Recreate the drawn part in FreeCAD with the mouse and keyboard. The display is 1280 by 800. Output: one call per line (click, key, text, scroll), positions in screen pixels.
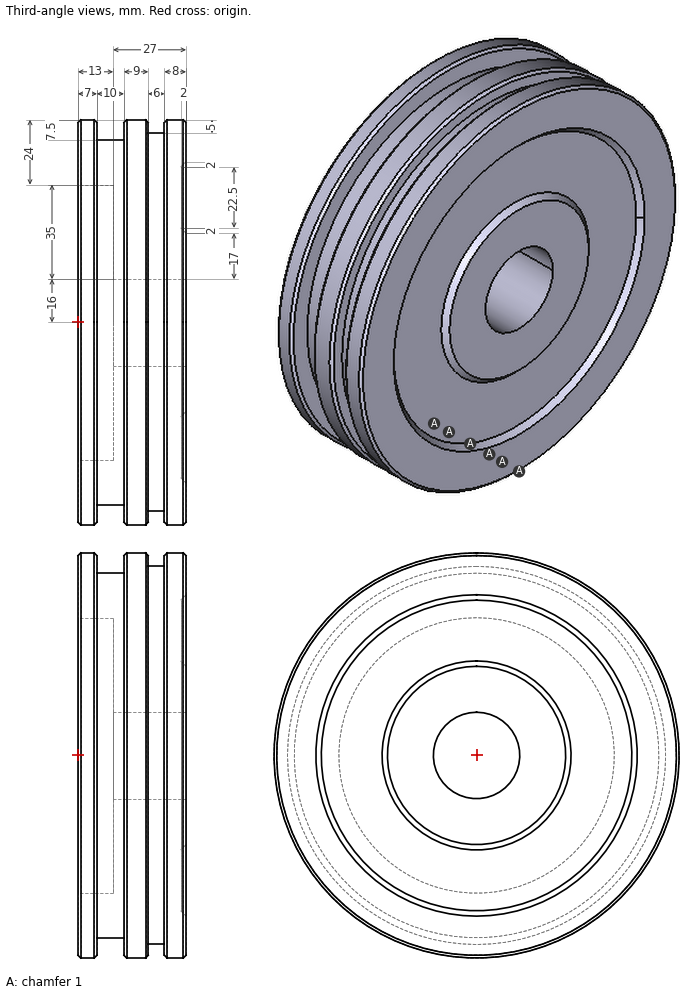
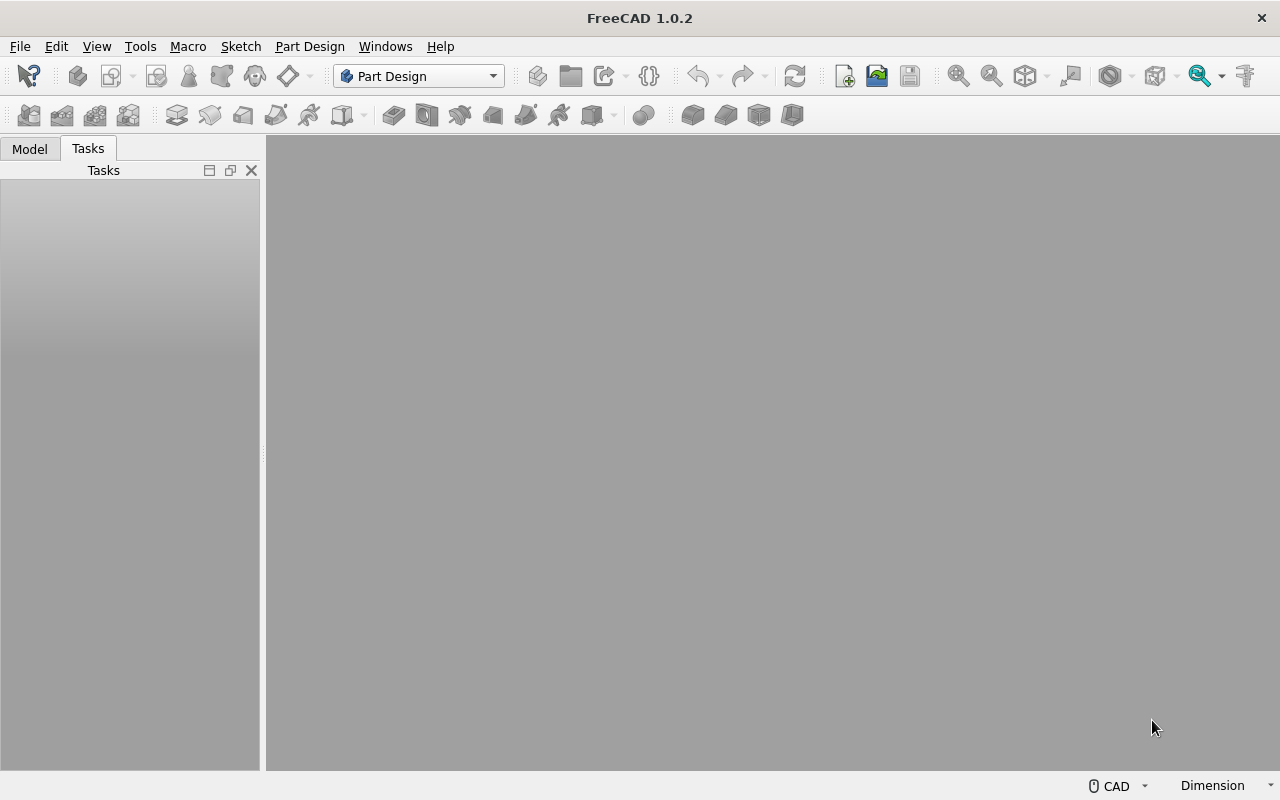
click(844, 76)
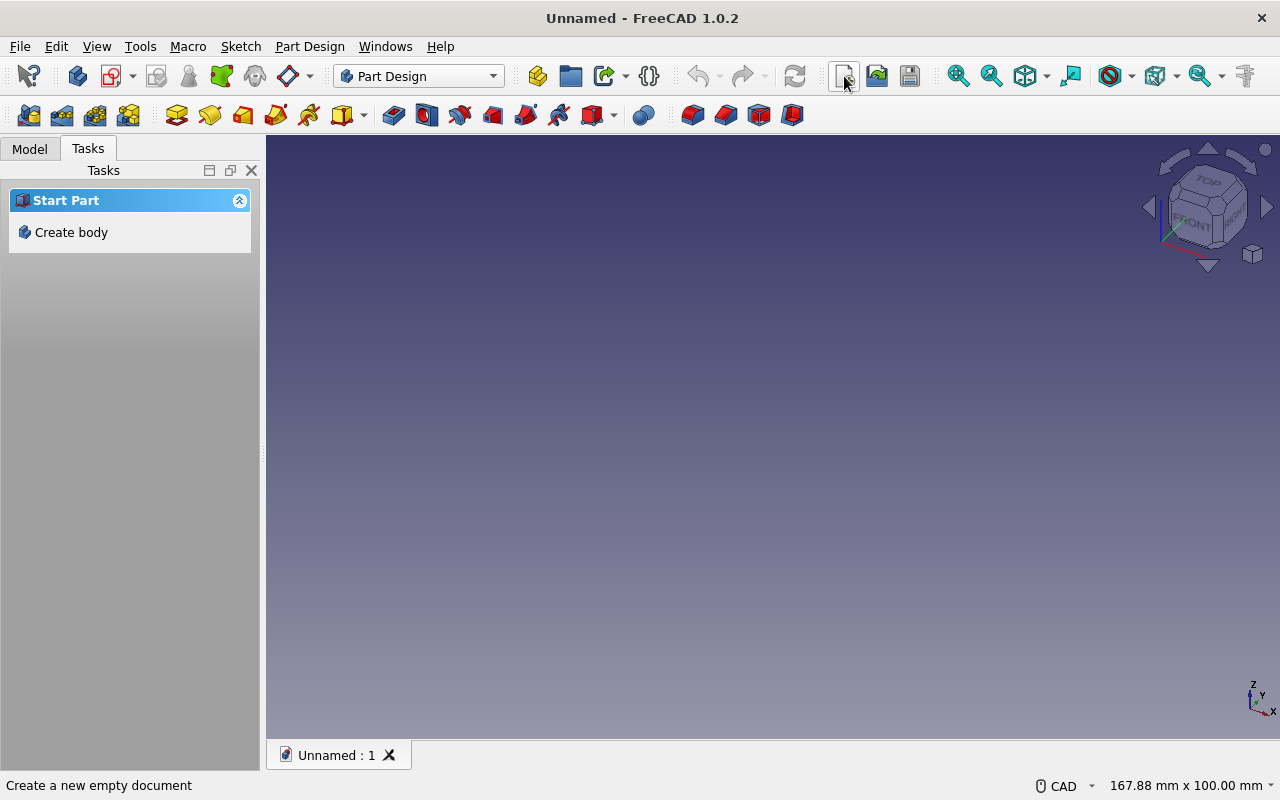
click(110, 76)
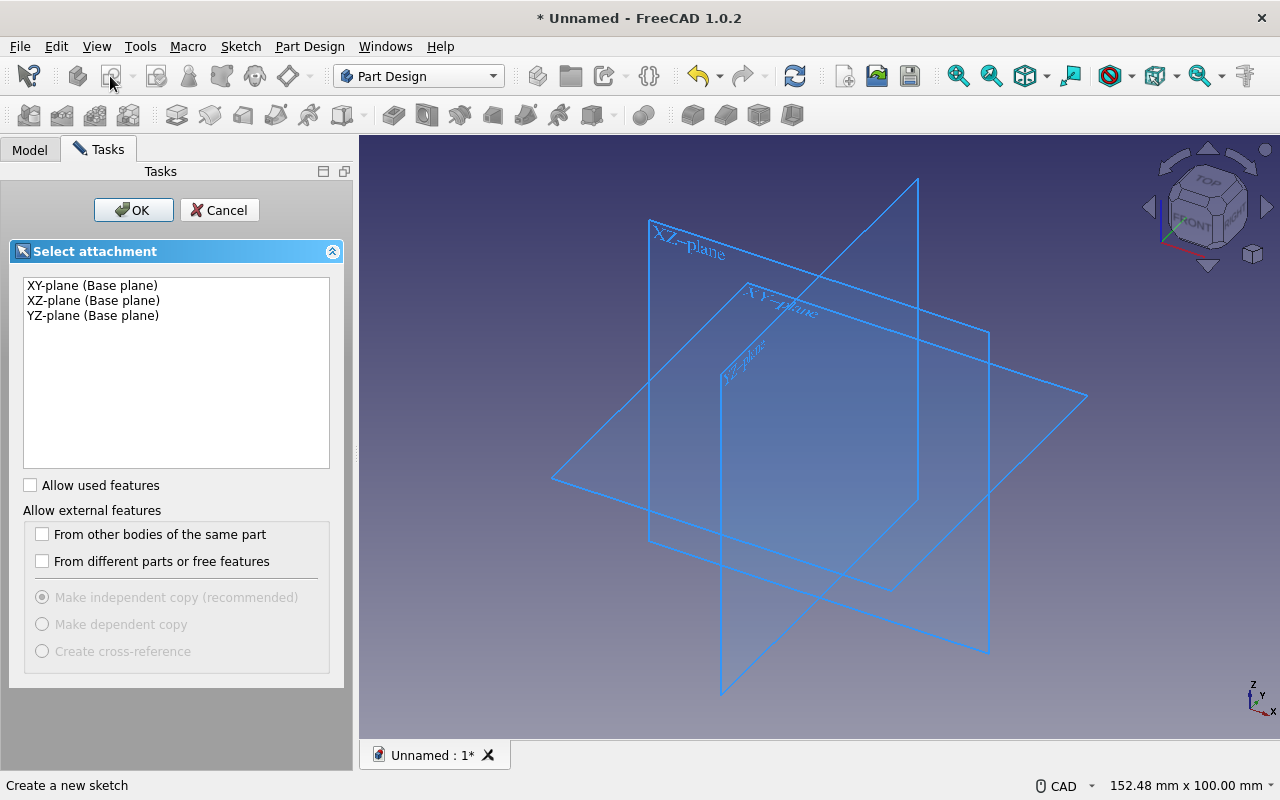
click(84, 286)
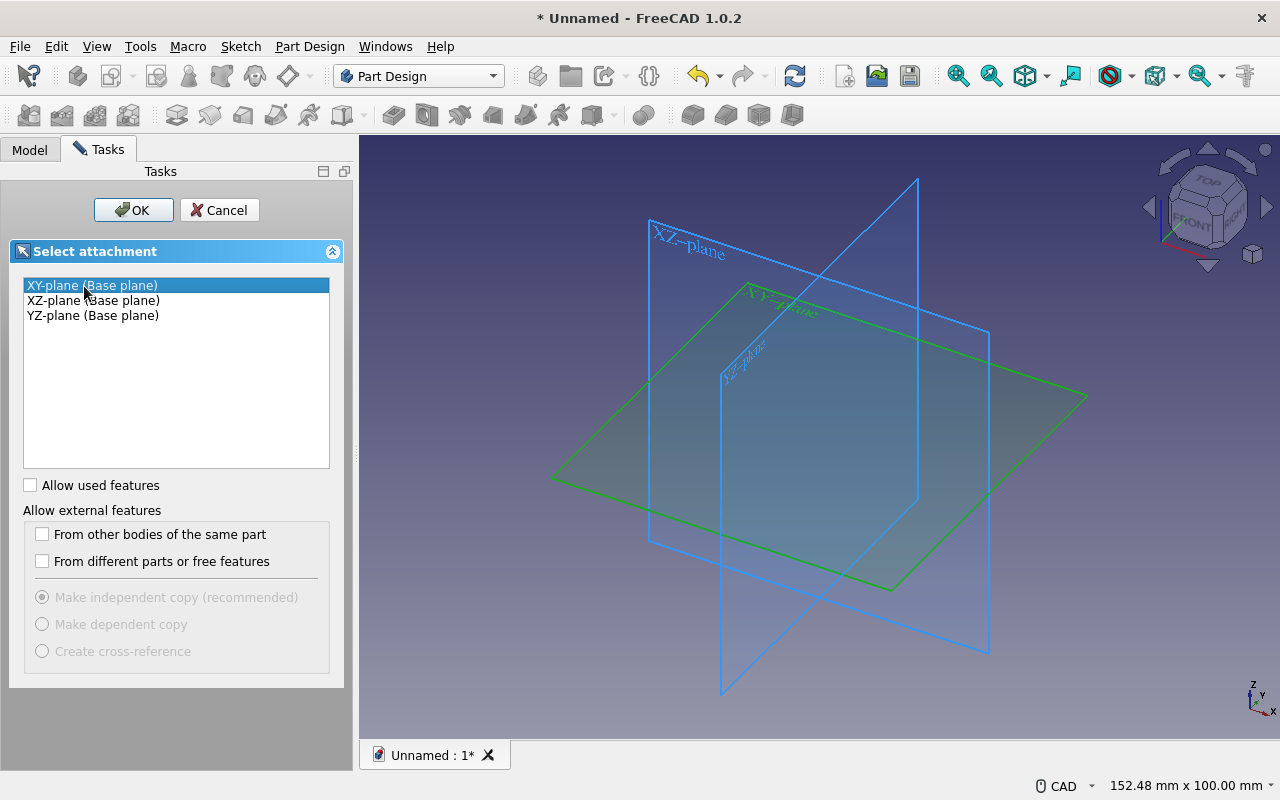
click(134, 210)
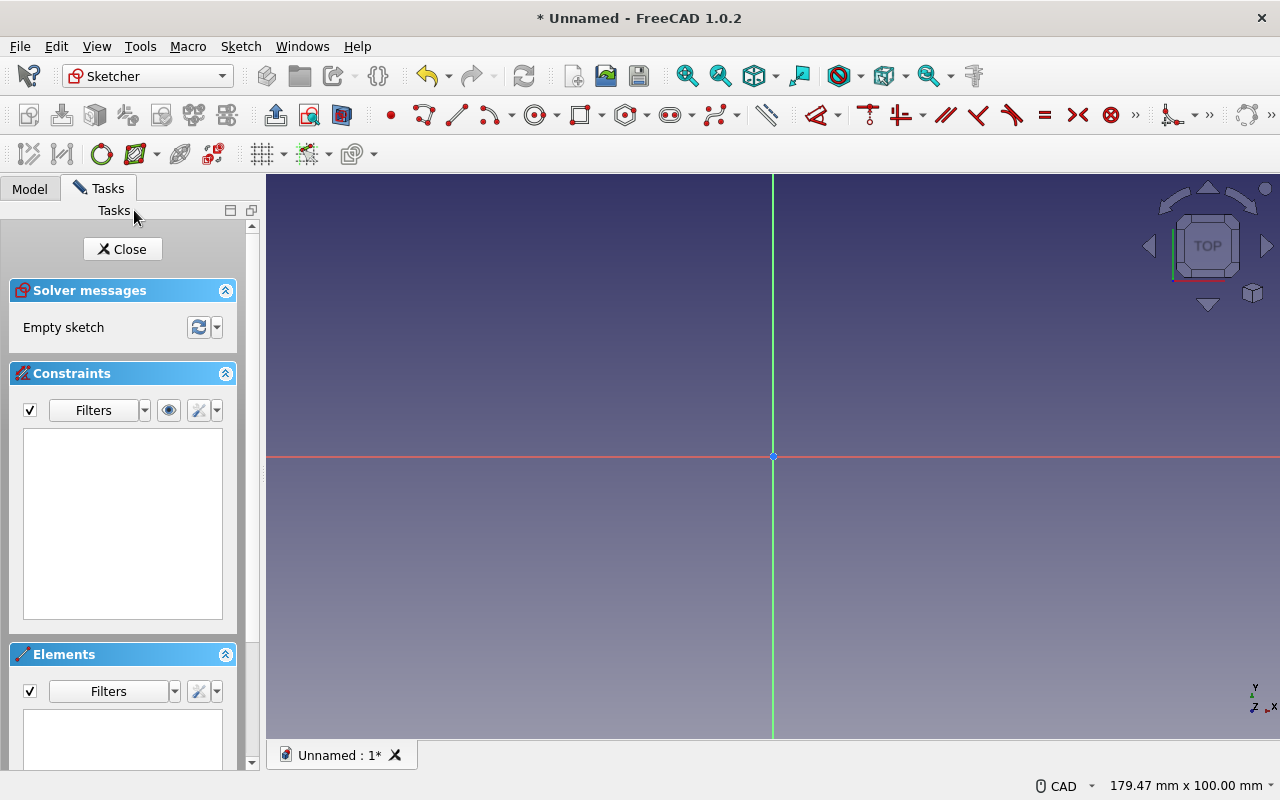
scroll(335, 711, down, 2)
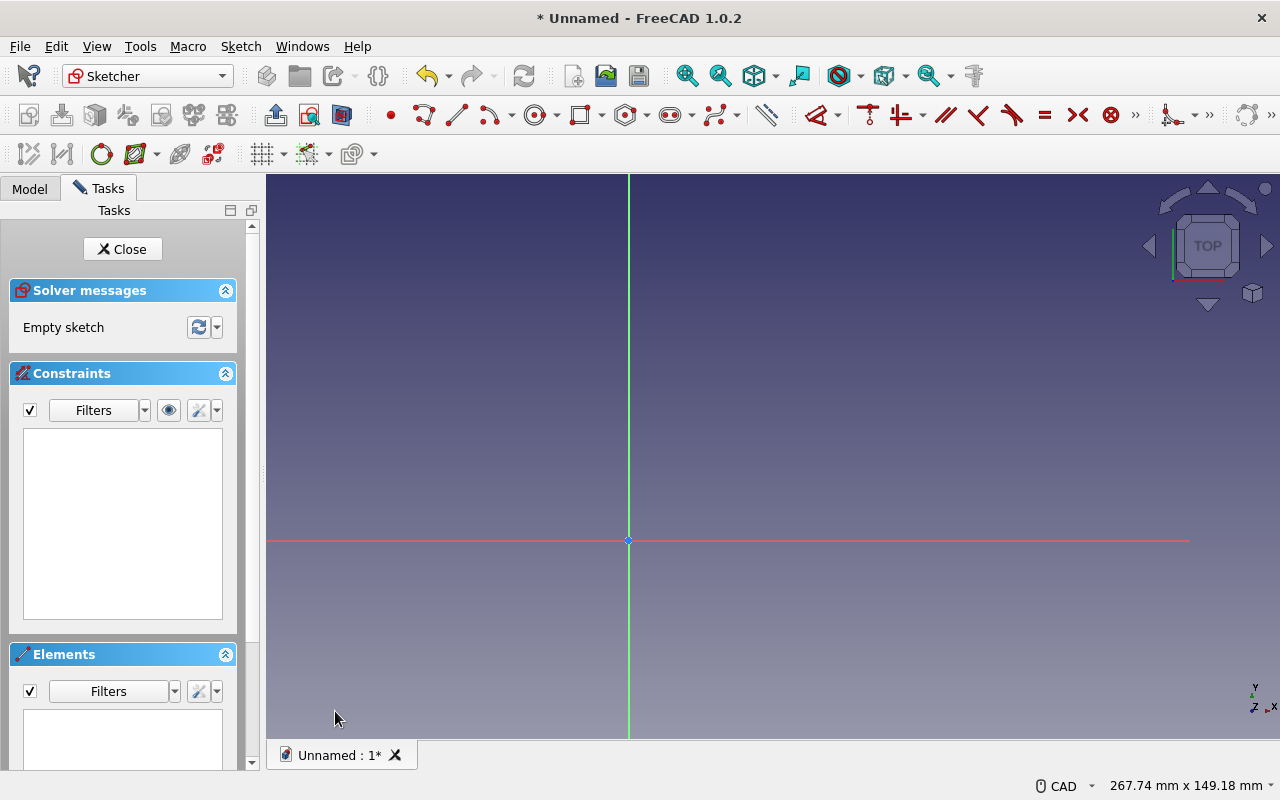
click(424, 116)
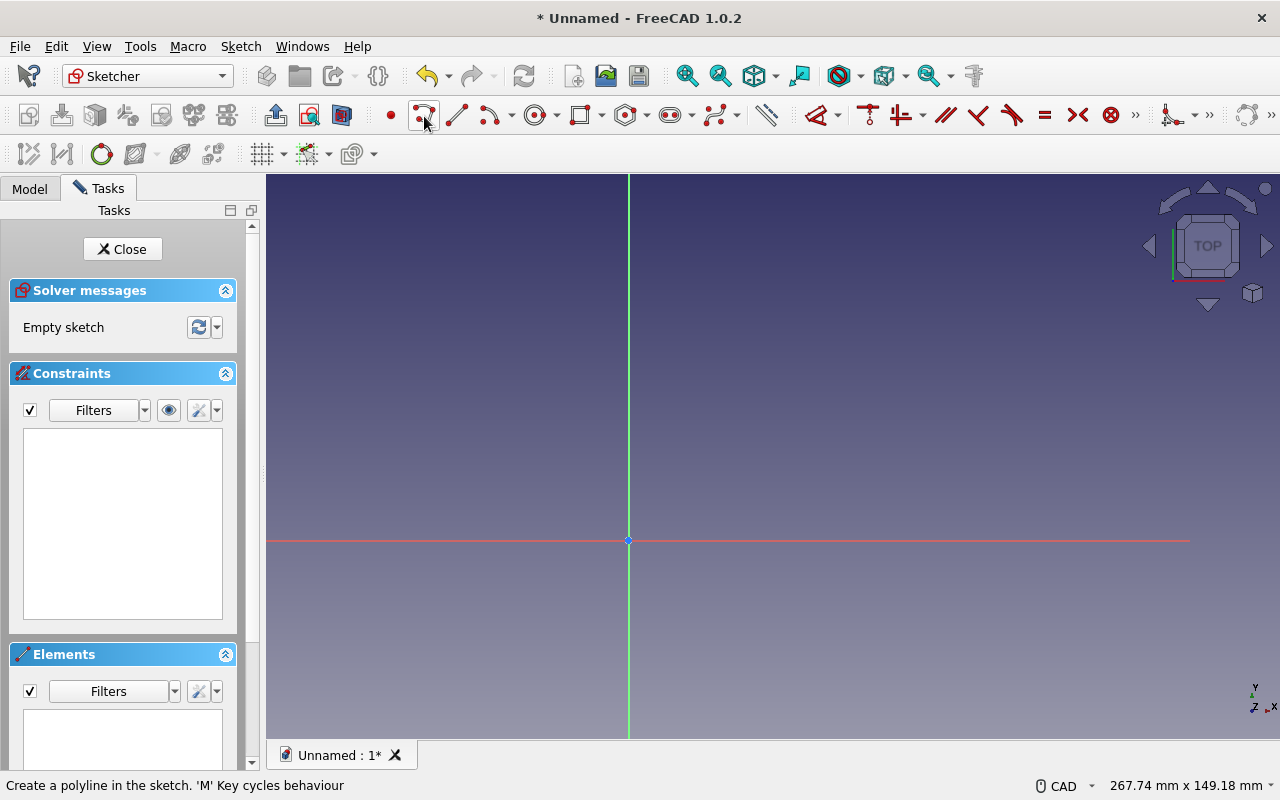
click(678, 480)
click(780, 480)
click(780, 416)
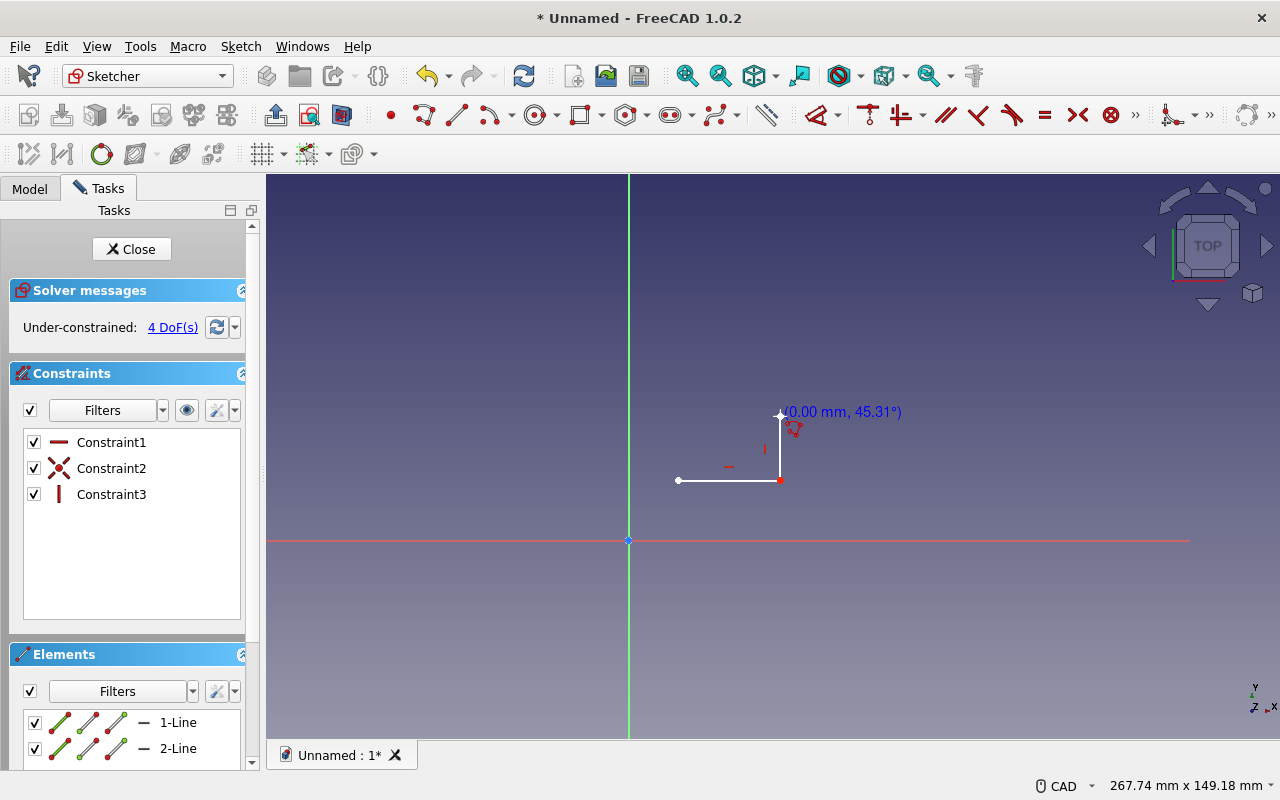
scroll(773, 408, up, 2)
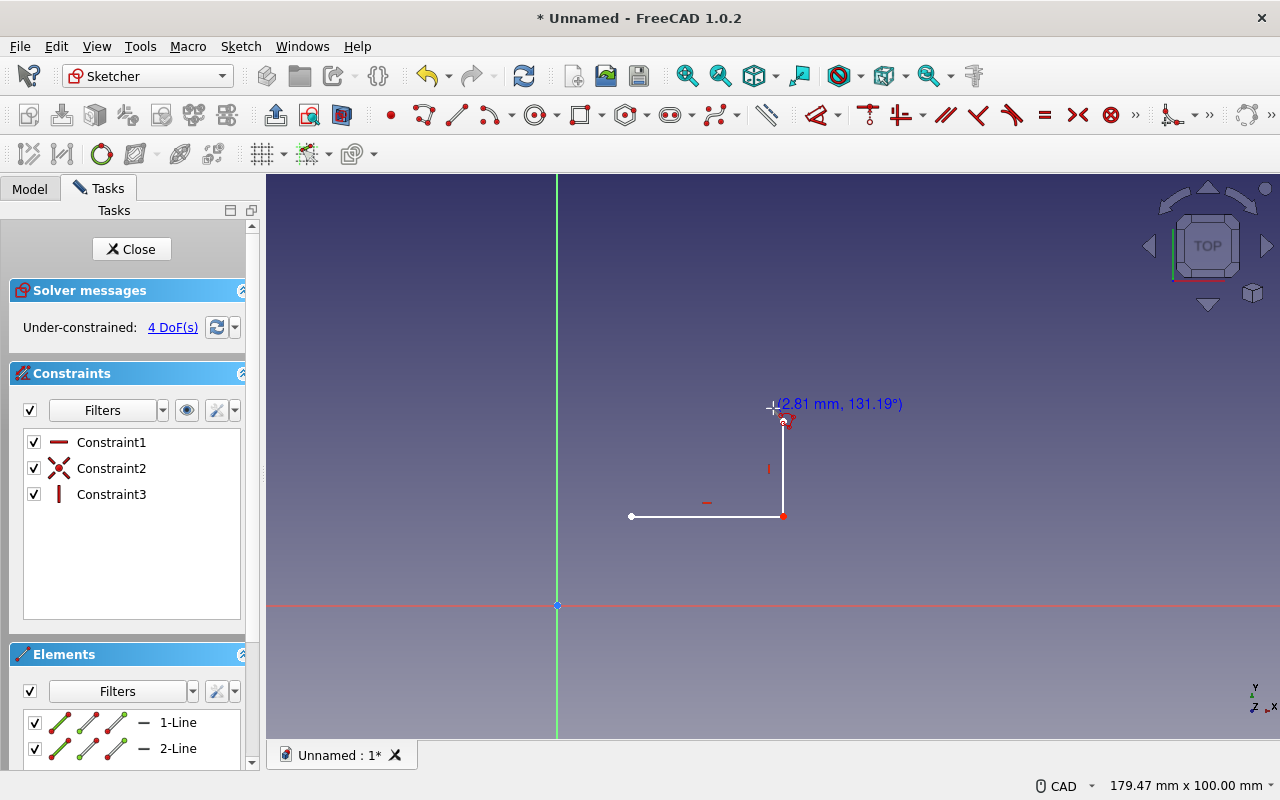
click(772, 408)
click(772, 281)
click(783, 270)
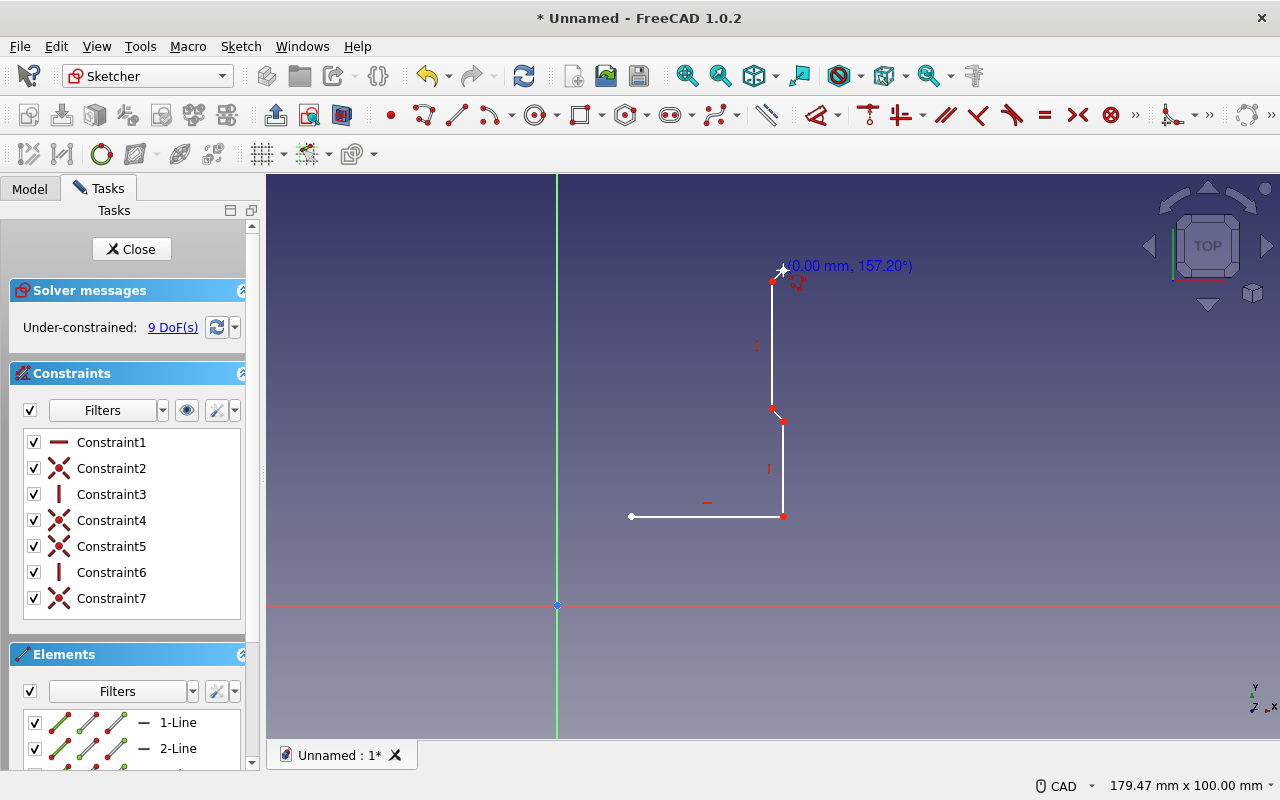
scroll(859, 711, down, 1)